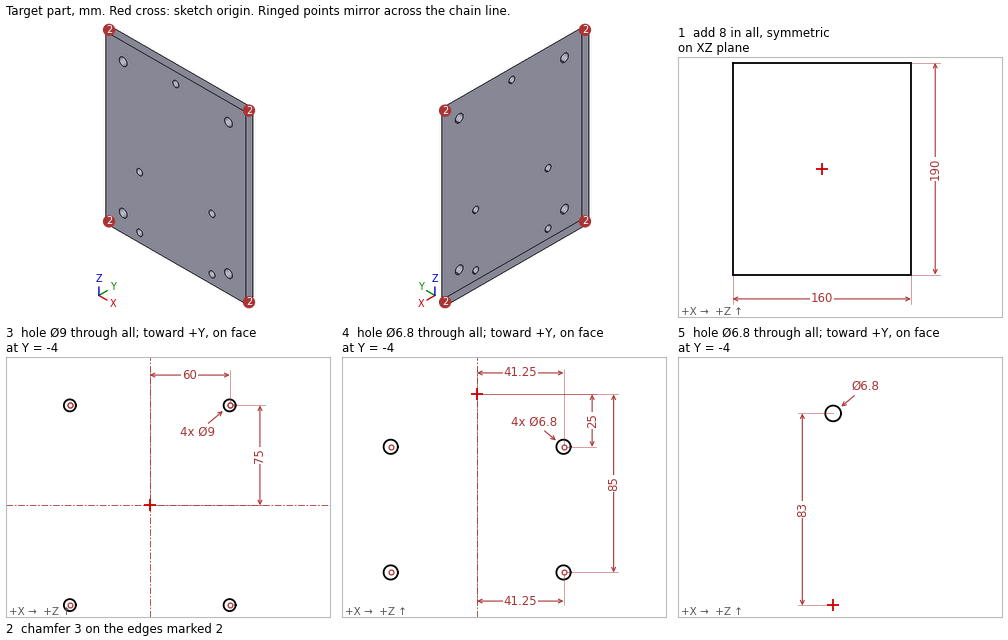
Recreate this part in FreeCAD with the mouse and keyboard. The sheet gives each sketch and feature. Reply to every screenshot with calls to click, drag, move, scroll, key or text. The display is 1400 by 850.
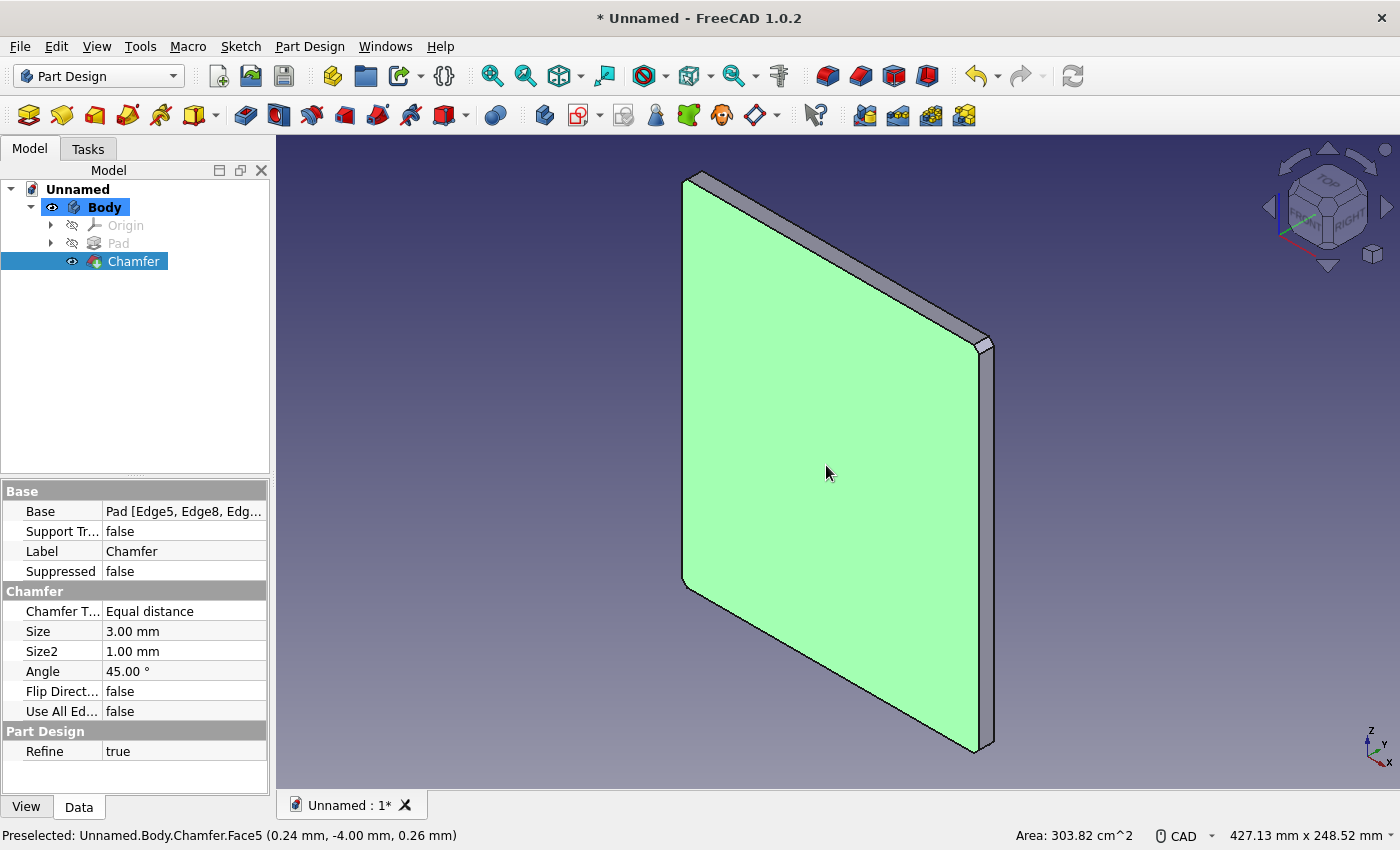
click(578, 116)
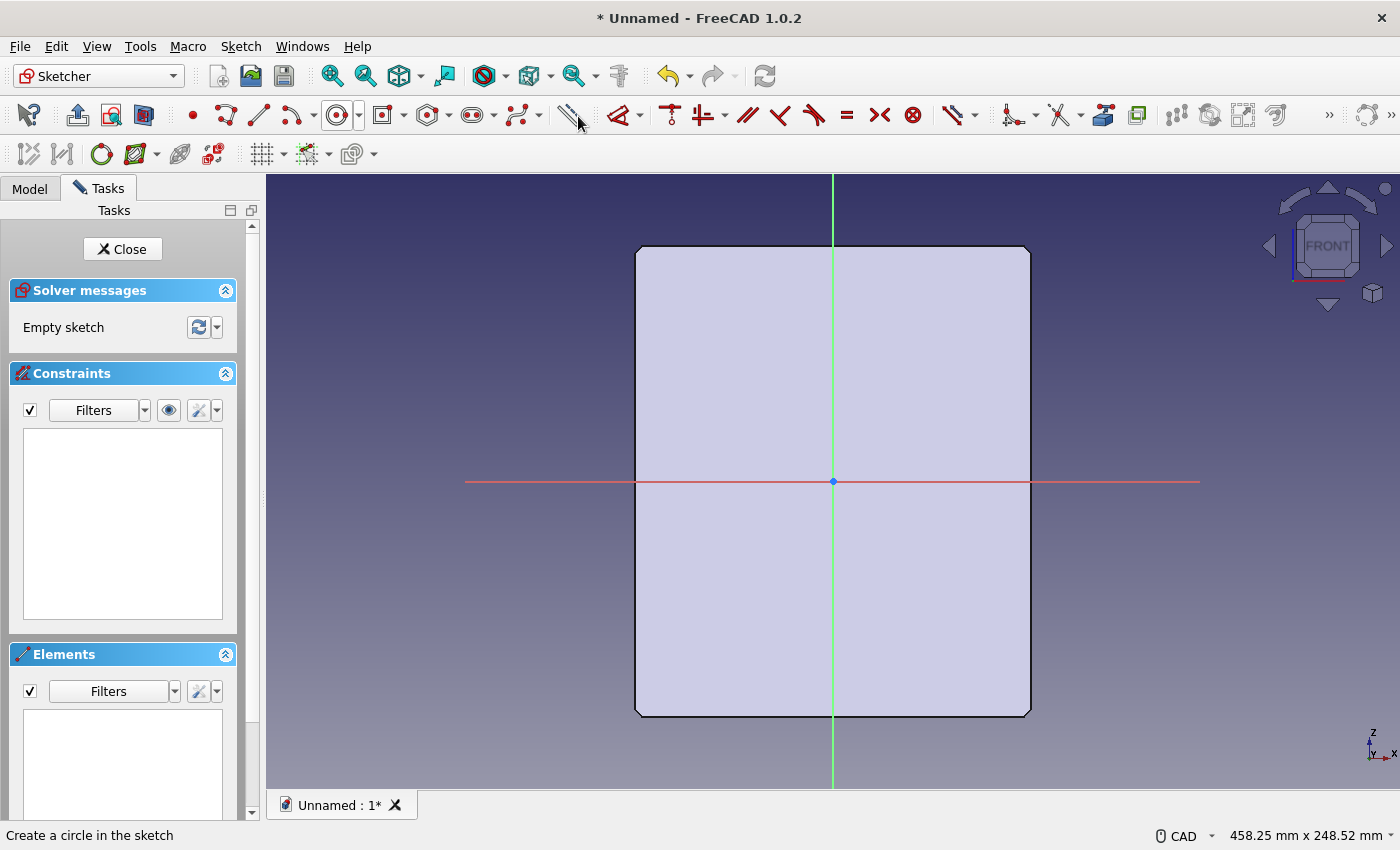
click(336, 116)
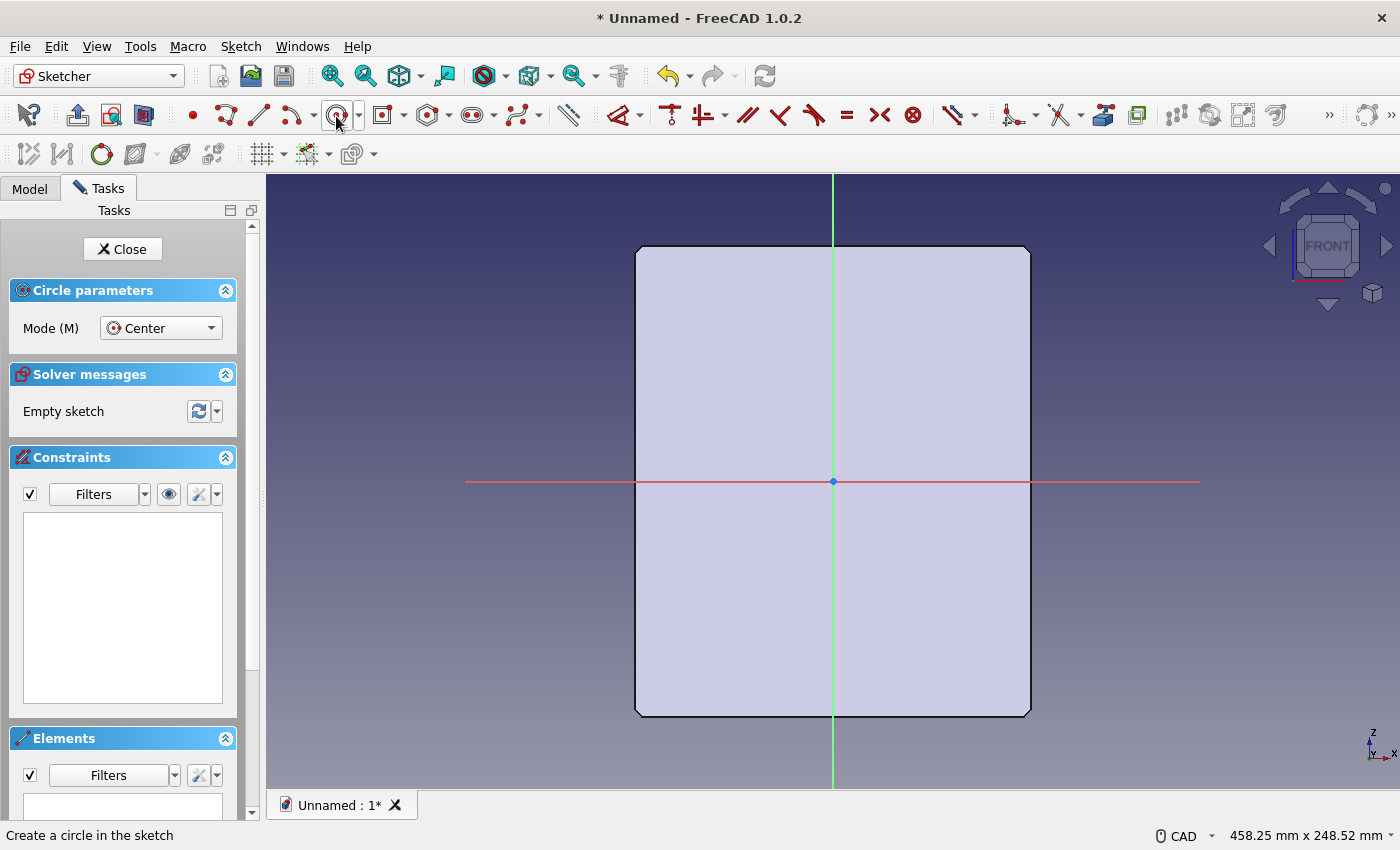
scroll(981, 296, up, 4)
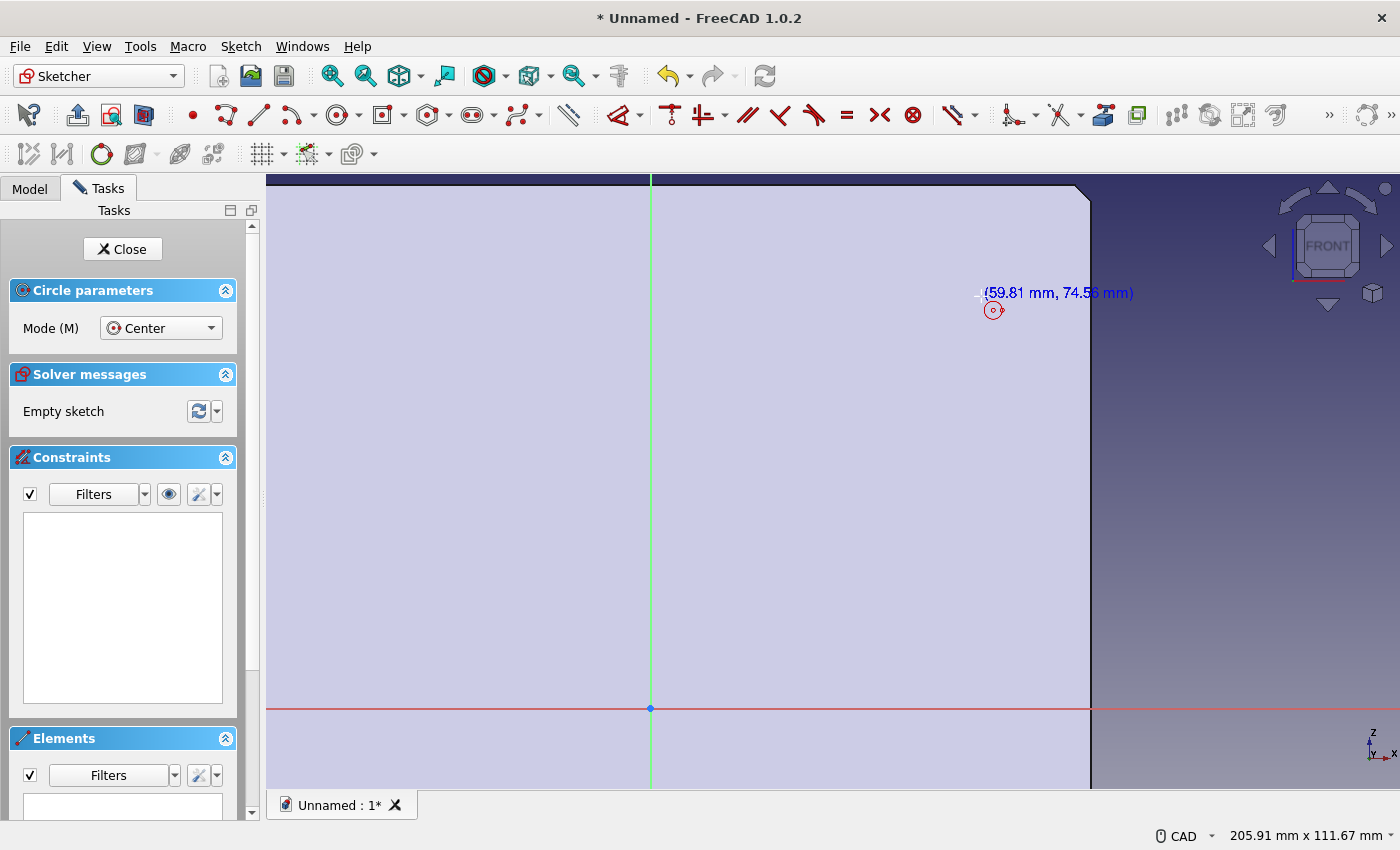
click(981, 296)
click(999, 278)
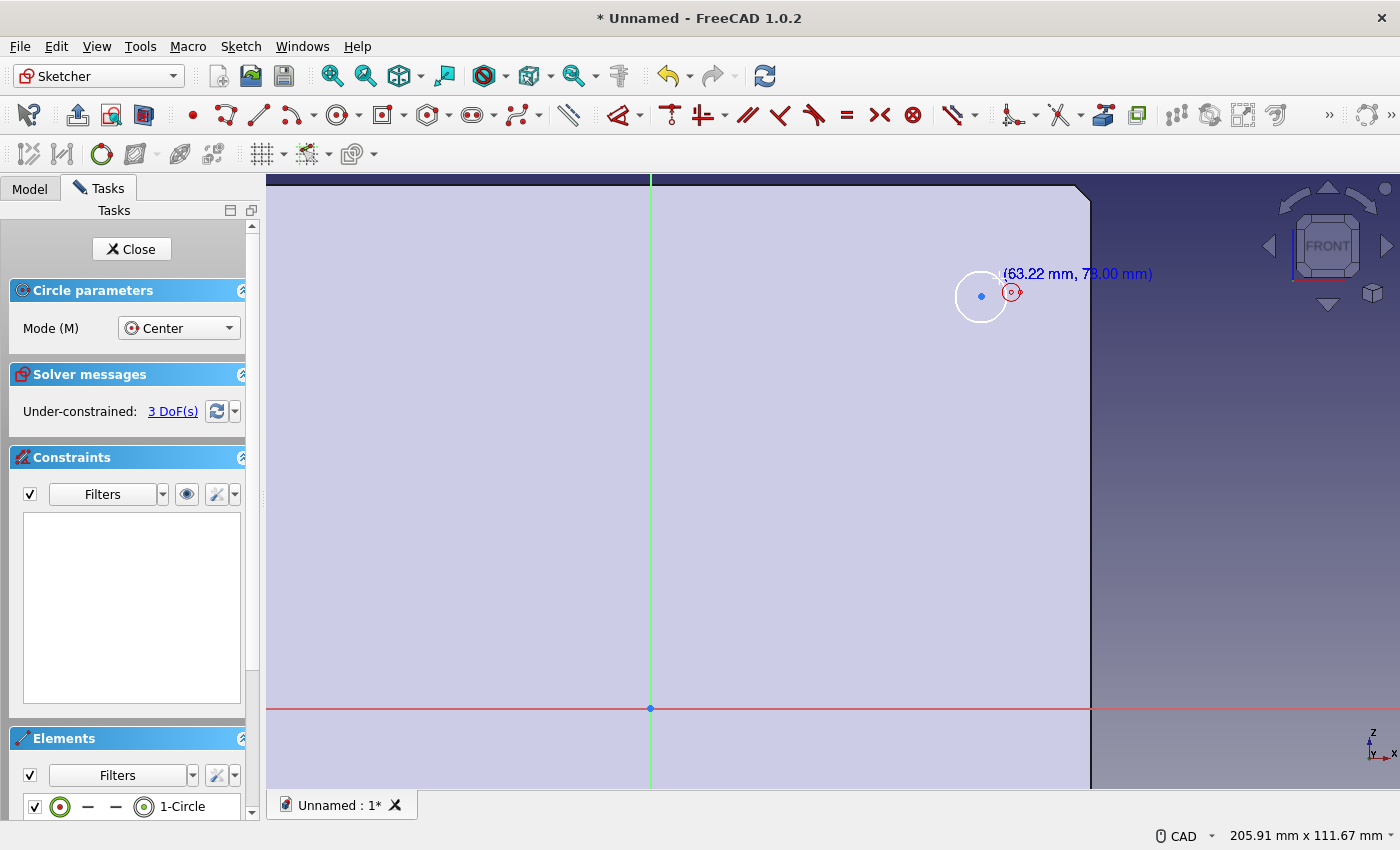
click(320, 296)
click(338, 278)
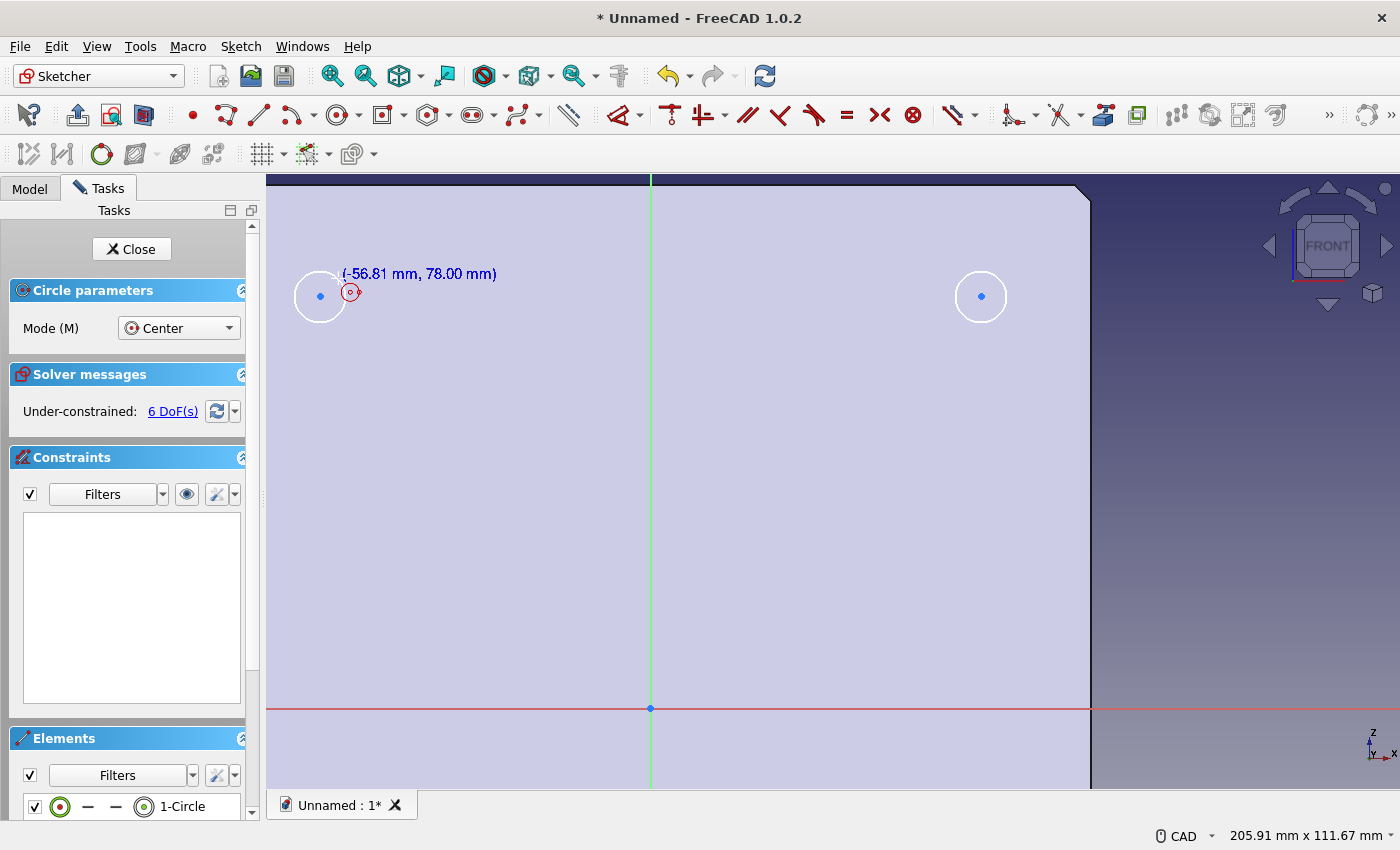
scroll(857, 296, down, 4)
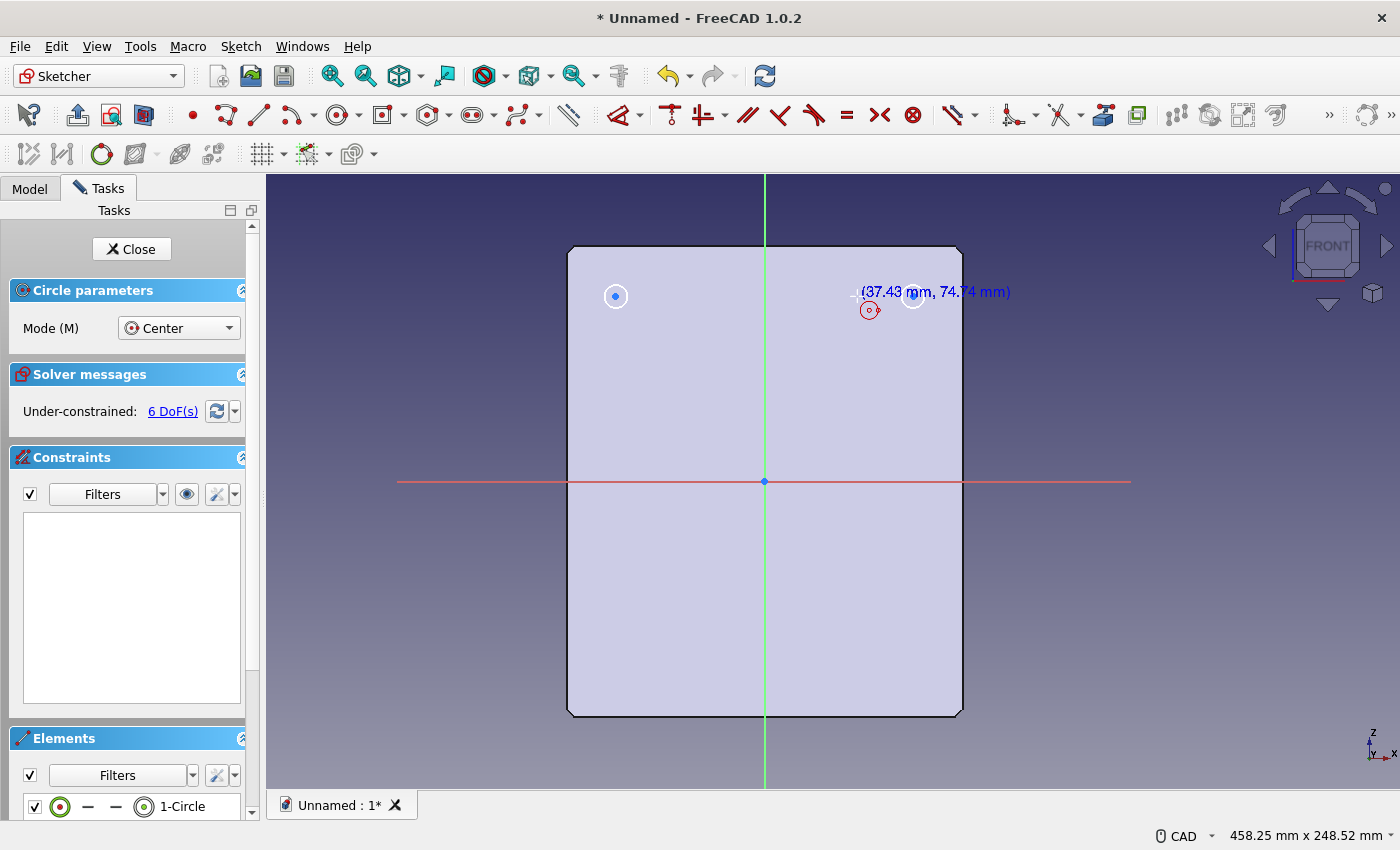
scroll(616, 667, up, 4)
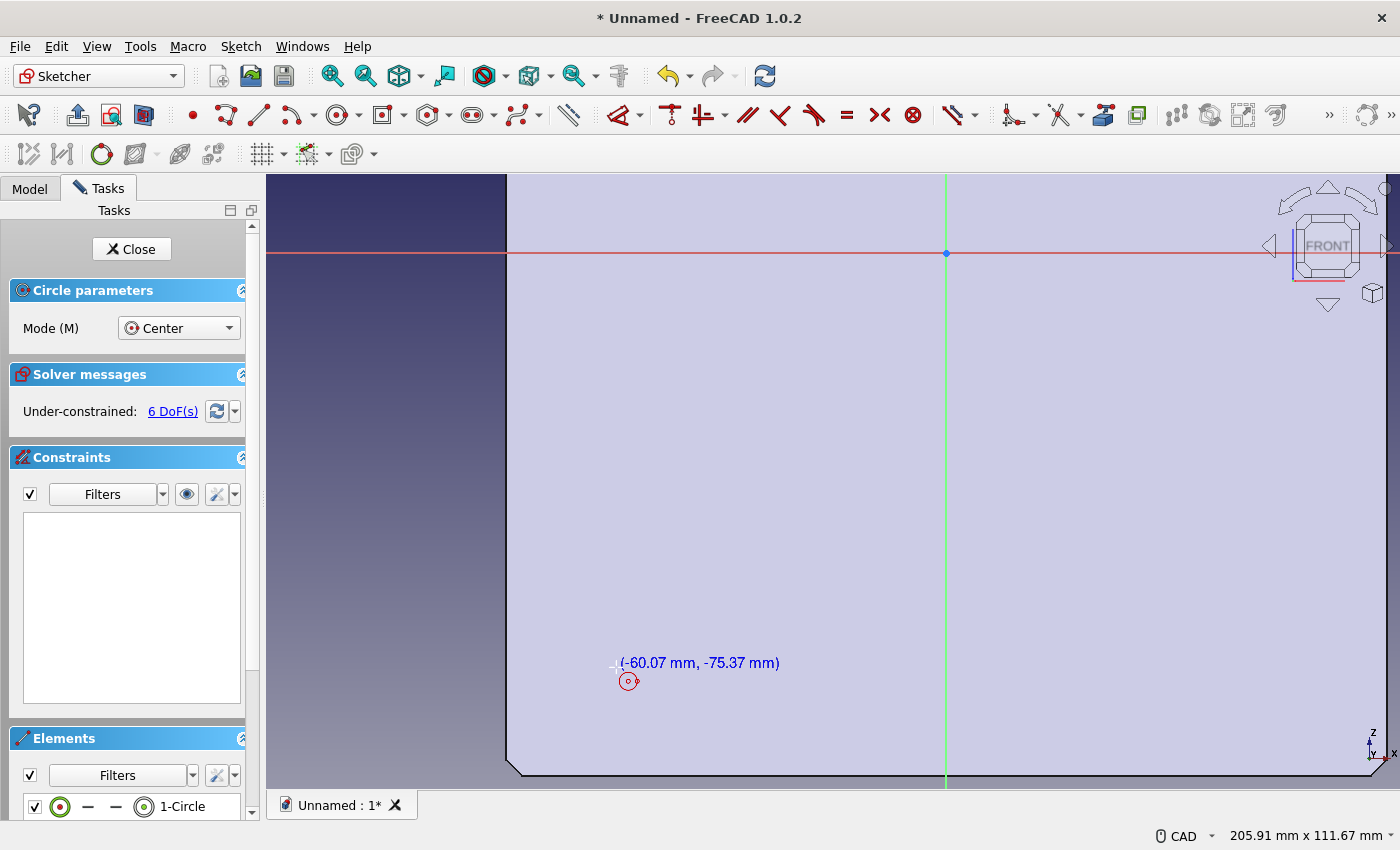
click(616, 666)
click(634, 649)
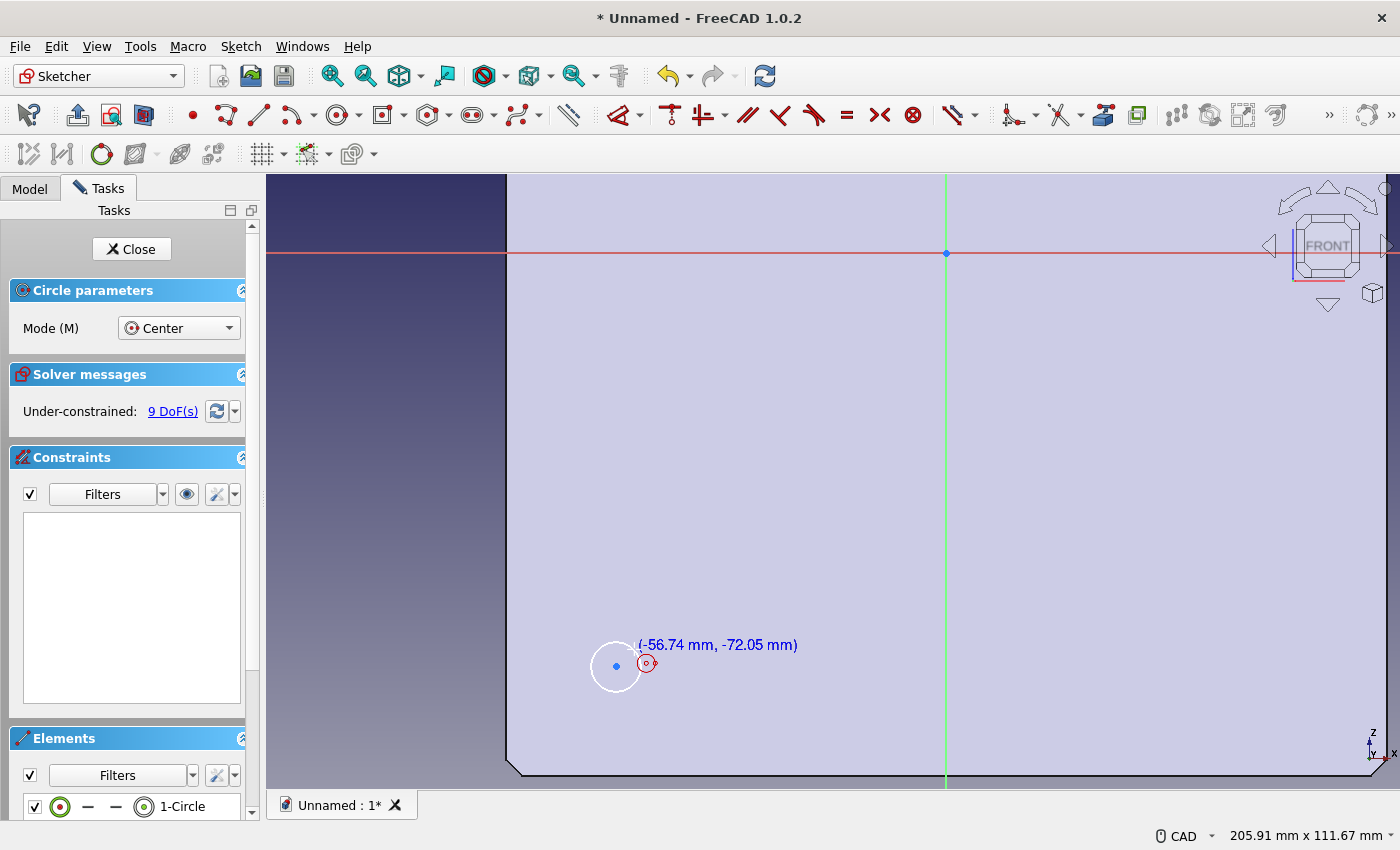
scroll(616, 668, down, 4)